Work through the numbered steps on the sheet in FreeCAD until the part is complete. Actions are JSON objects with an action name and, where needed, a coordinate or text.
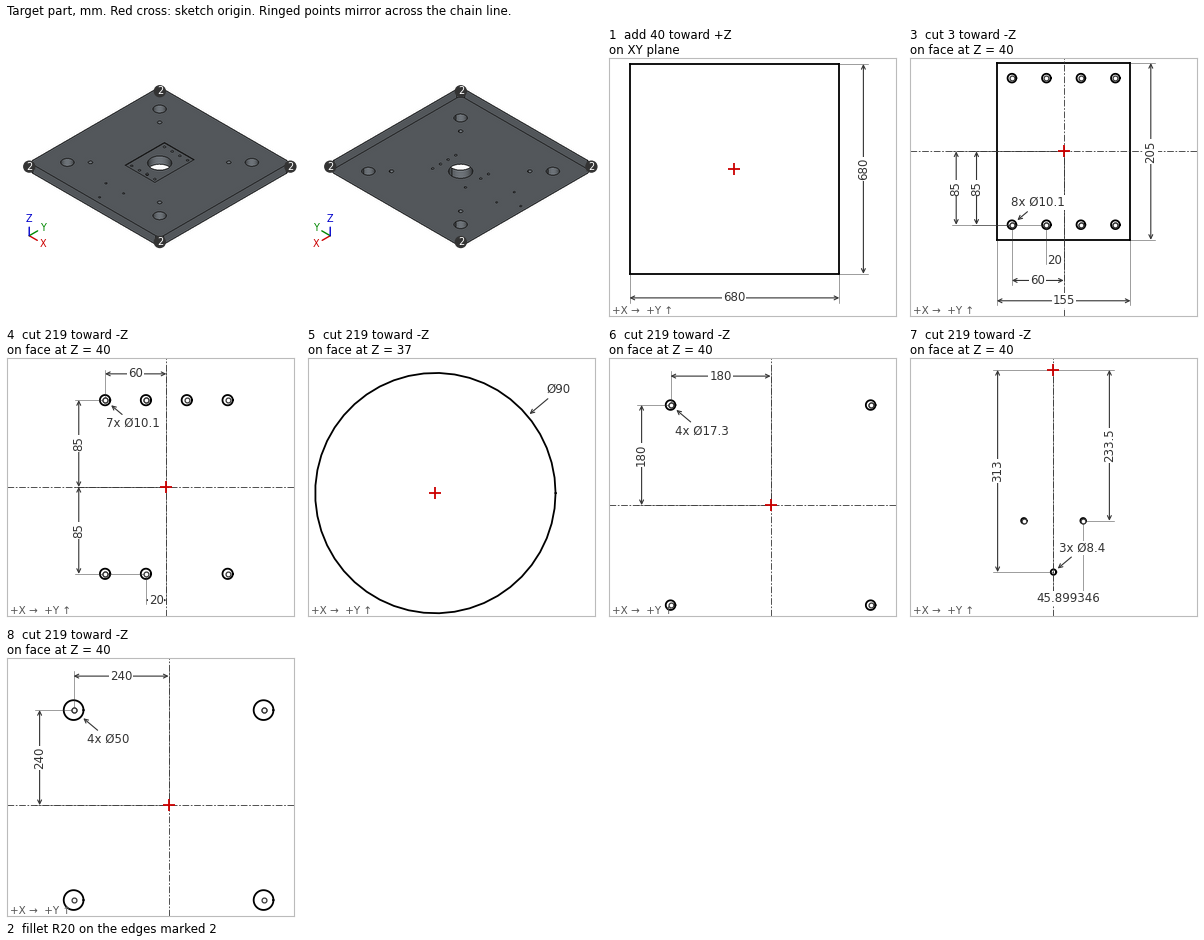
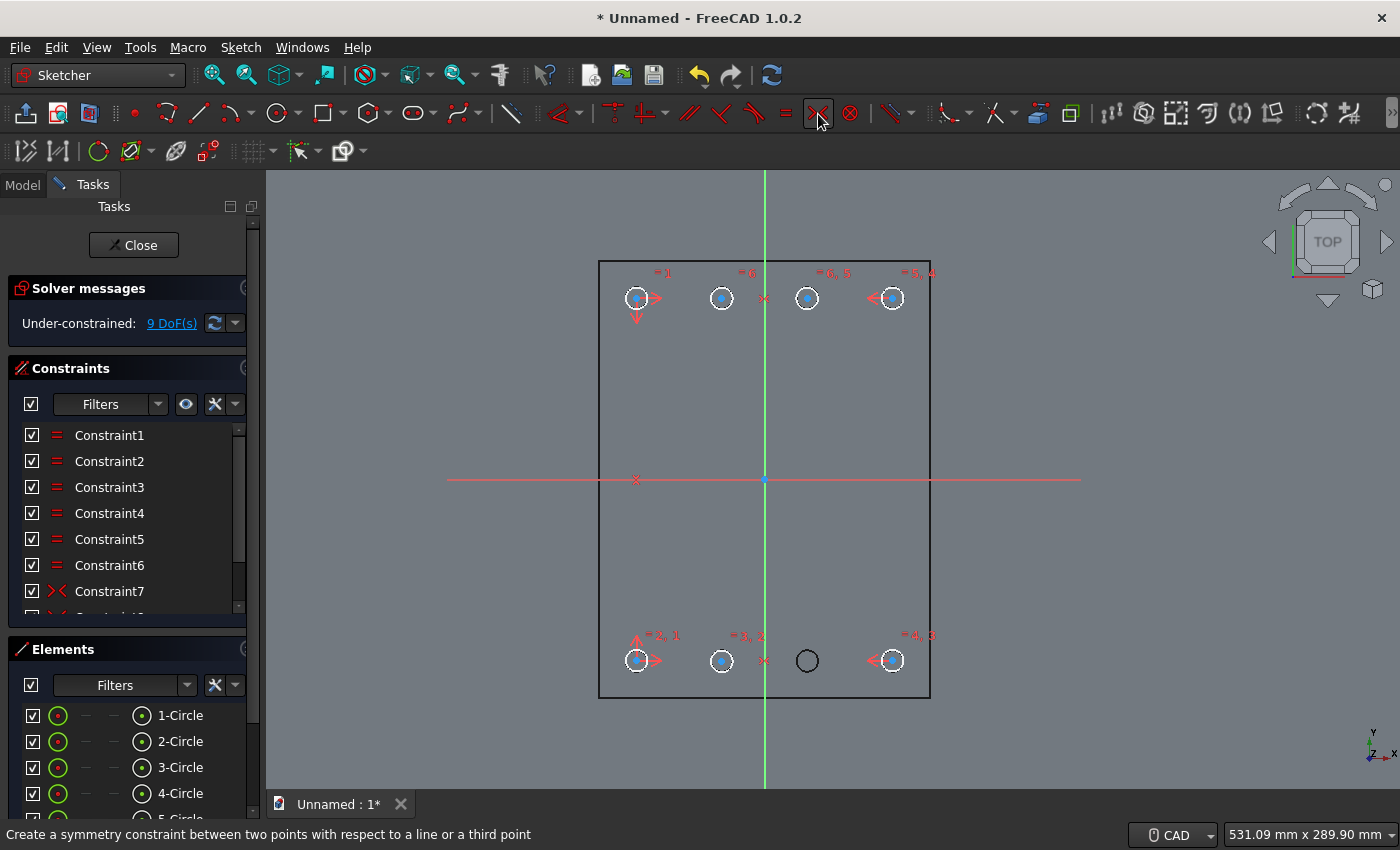
{"action": "left_click", "coordinate": [722, 661]}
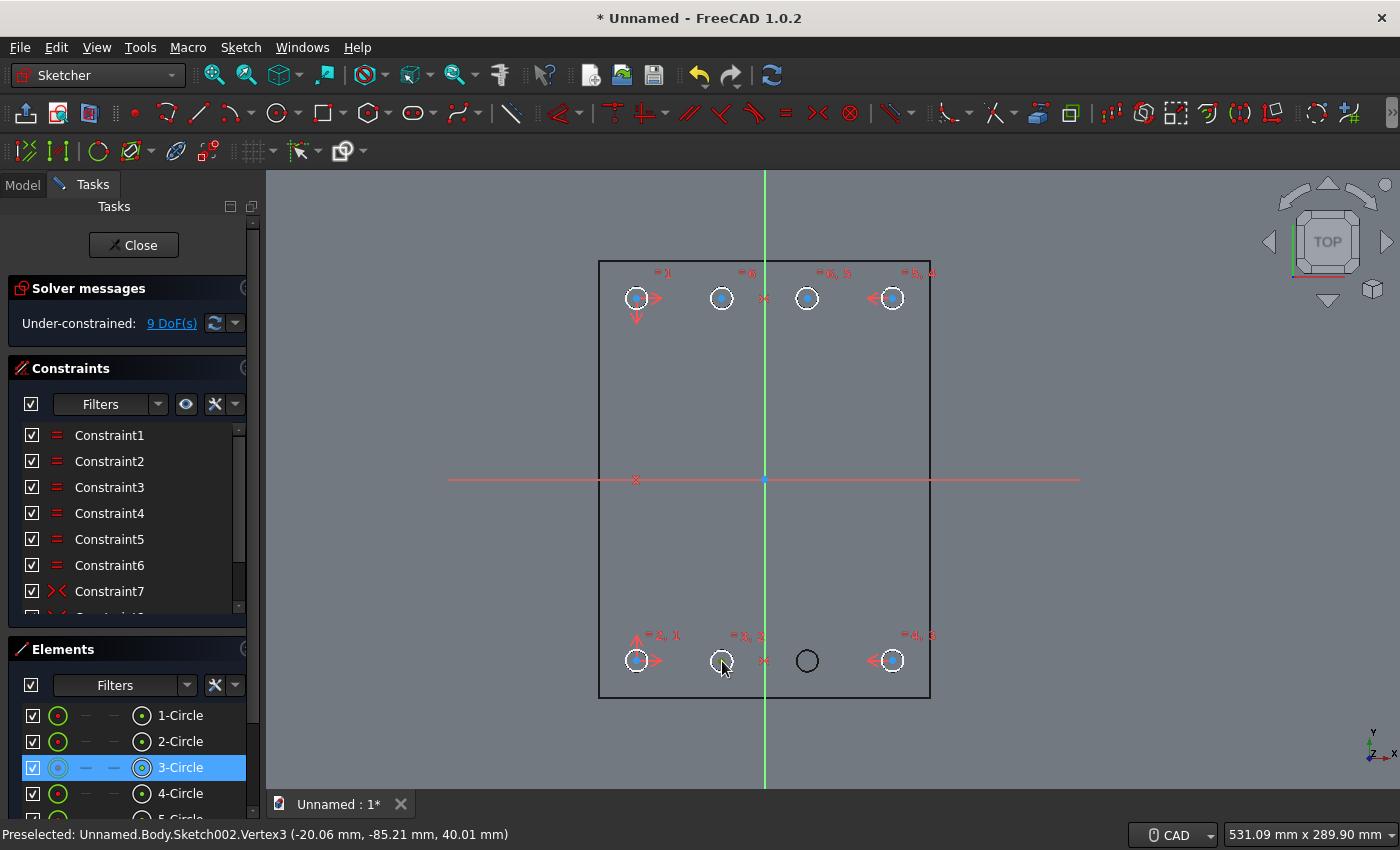
{"action": "left_click", "coordinate": [722, 299]}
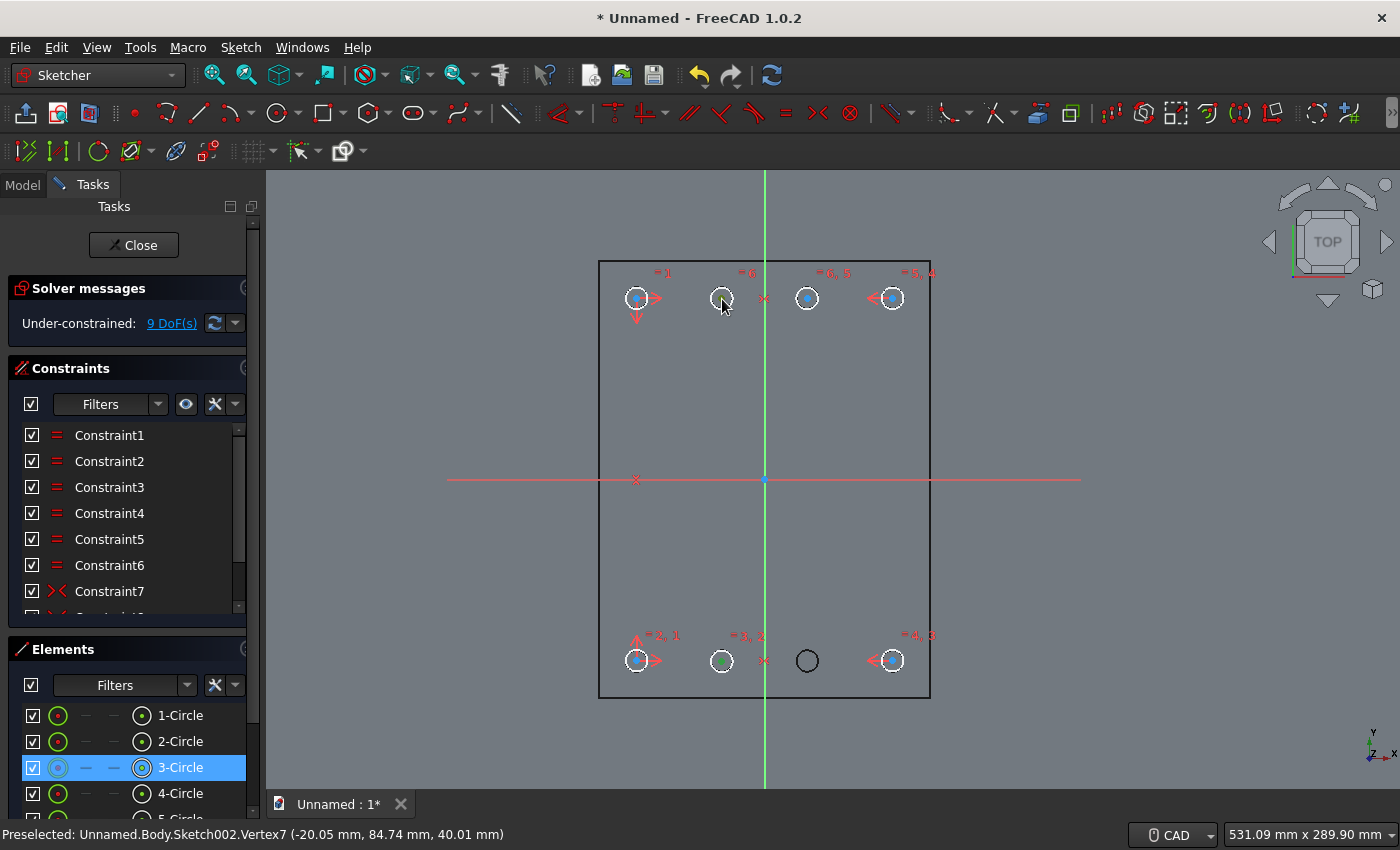
{"action": "left_click", "coordinate": [496, 480]}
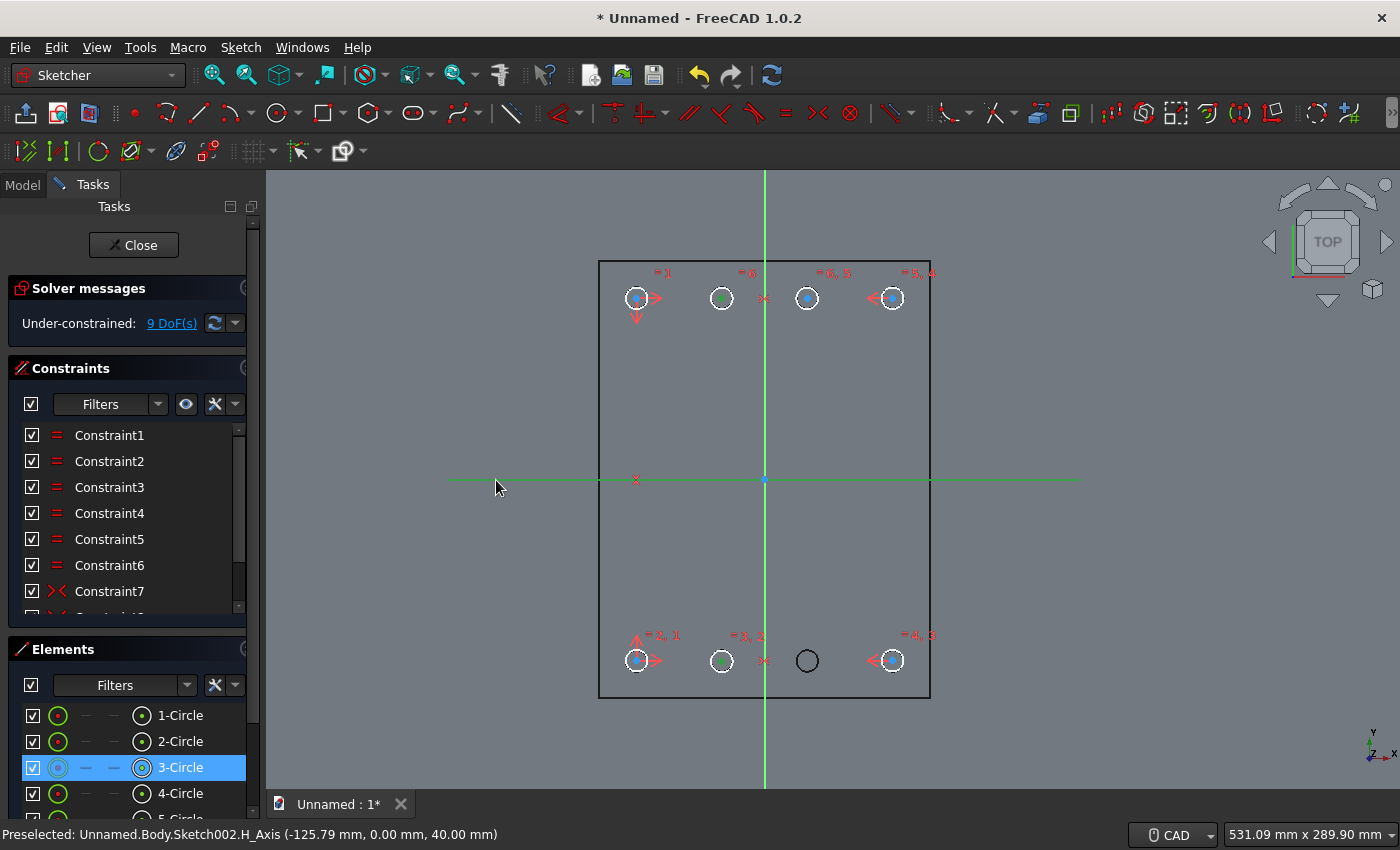
{"action": "left_click", "coordinate": [818, 114]}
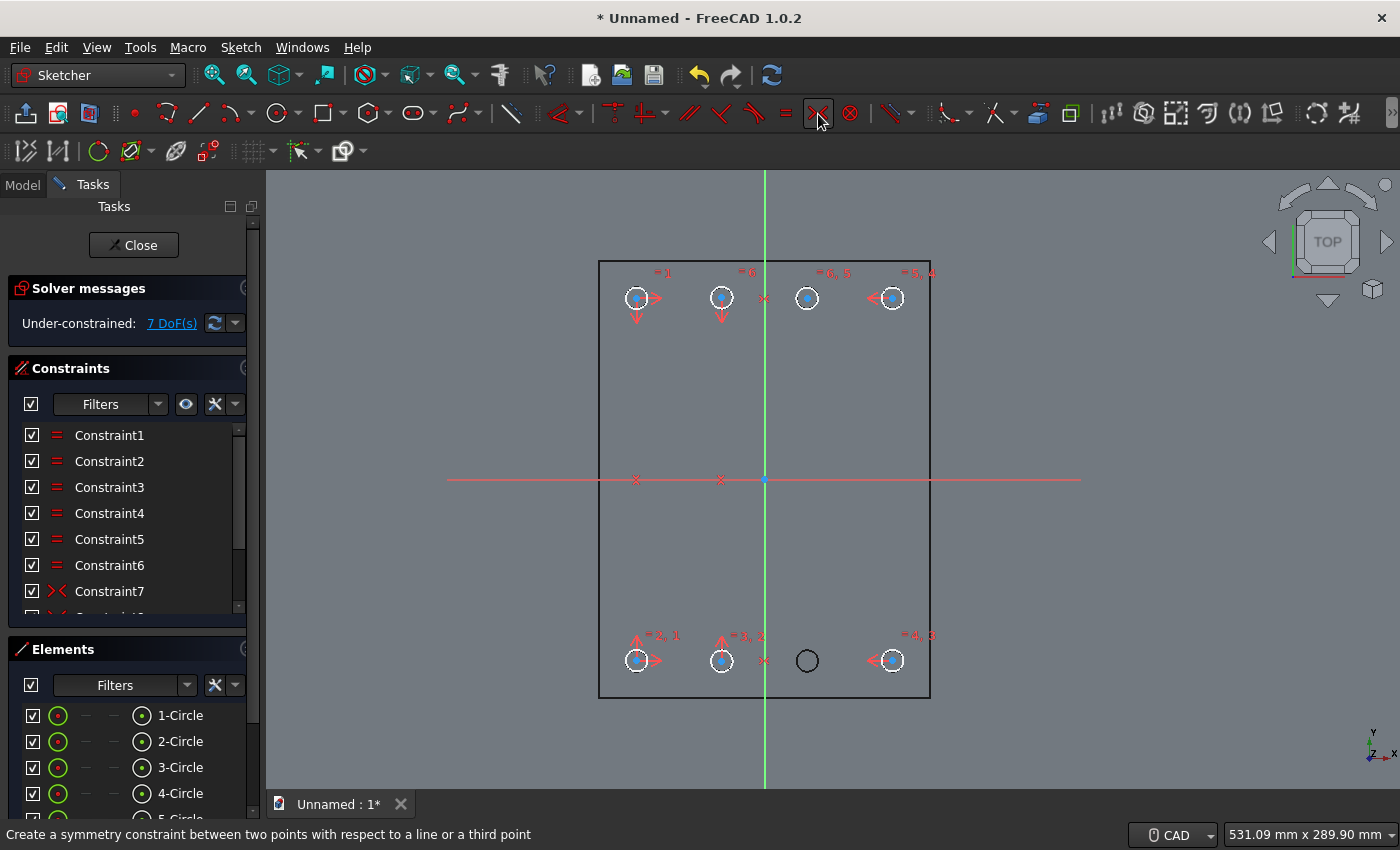
{"action": "left_click", "coordinate": [807, 299]}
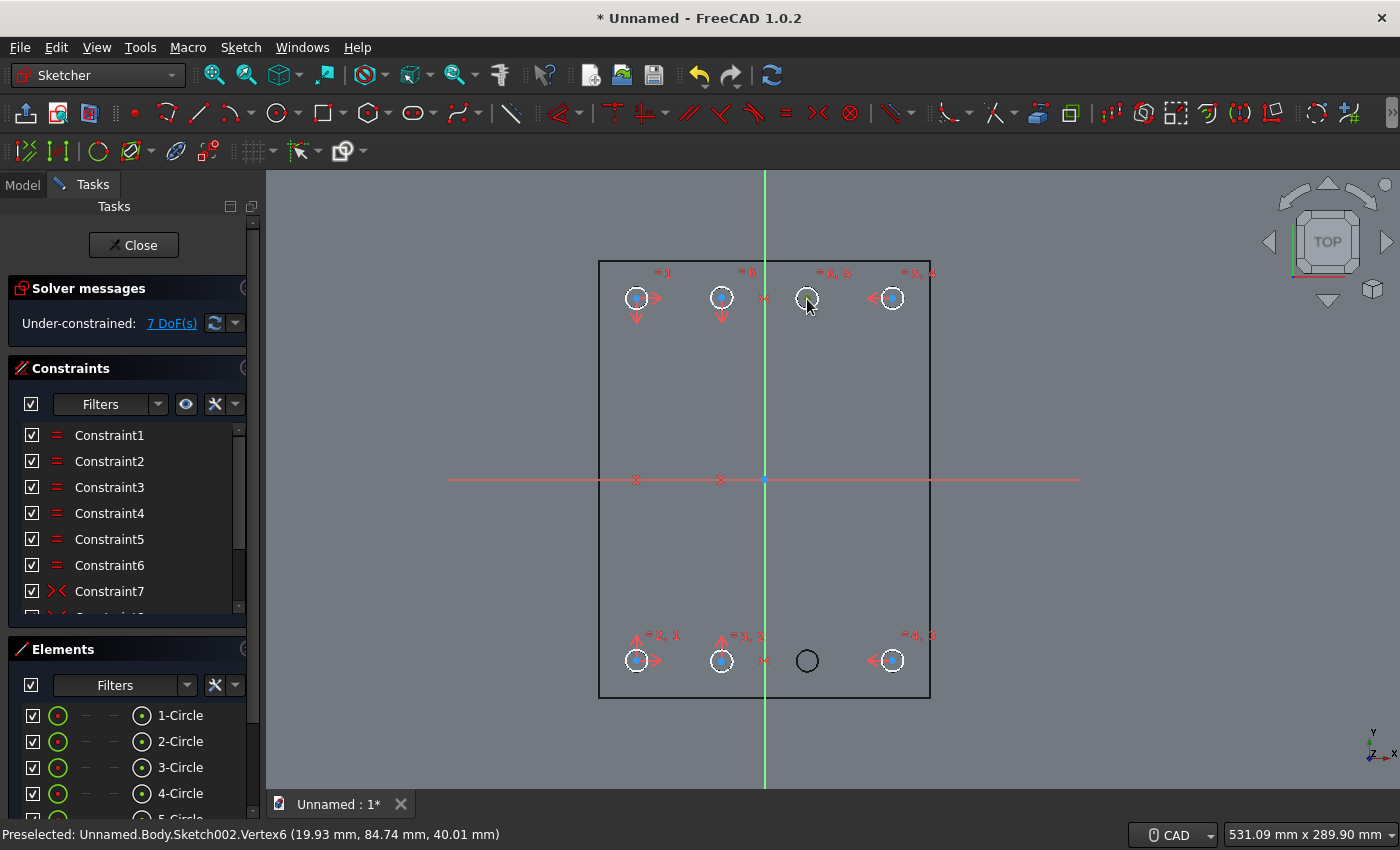
{"action": "left_click", "coordinate": [722, 298]}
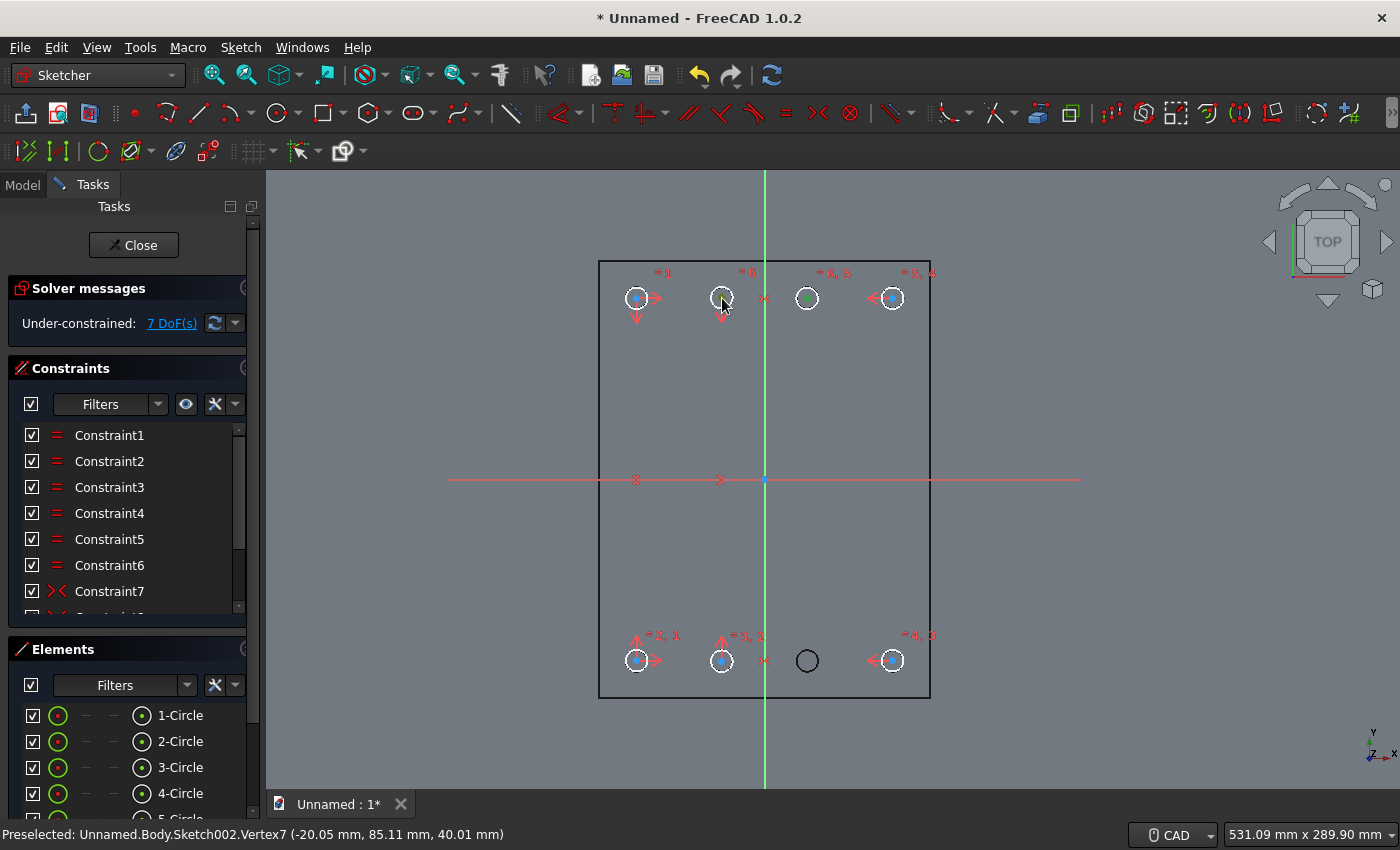
{"action": "left_click", "coordinate": [765, 721]}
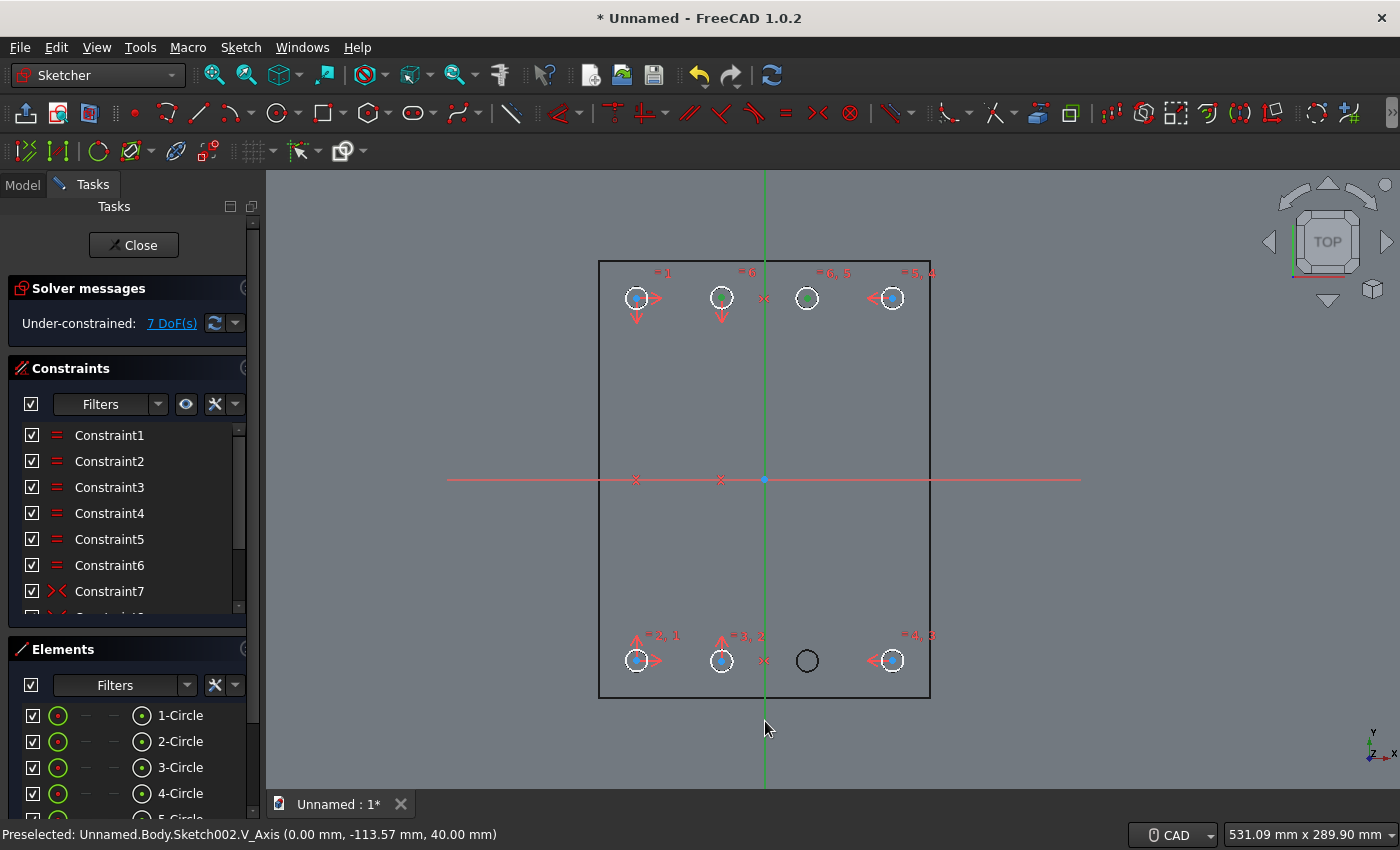
{"action": "left_click", "coordinate": [818, 114]}